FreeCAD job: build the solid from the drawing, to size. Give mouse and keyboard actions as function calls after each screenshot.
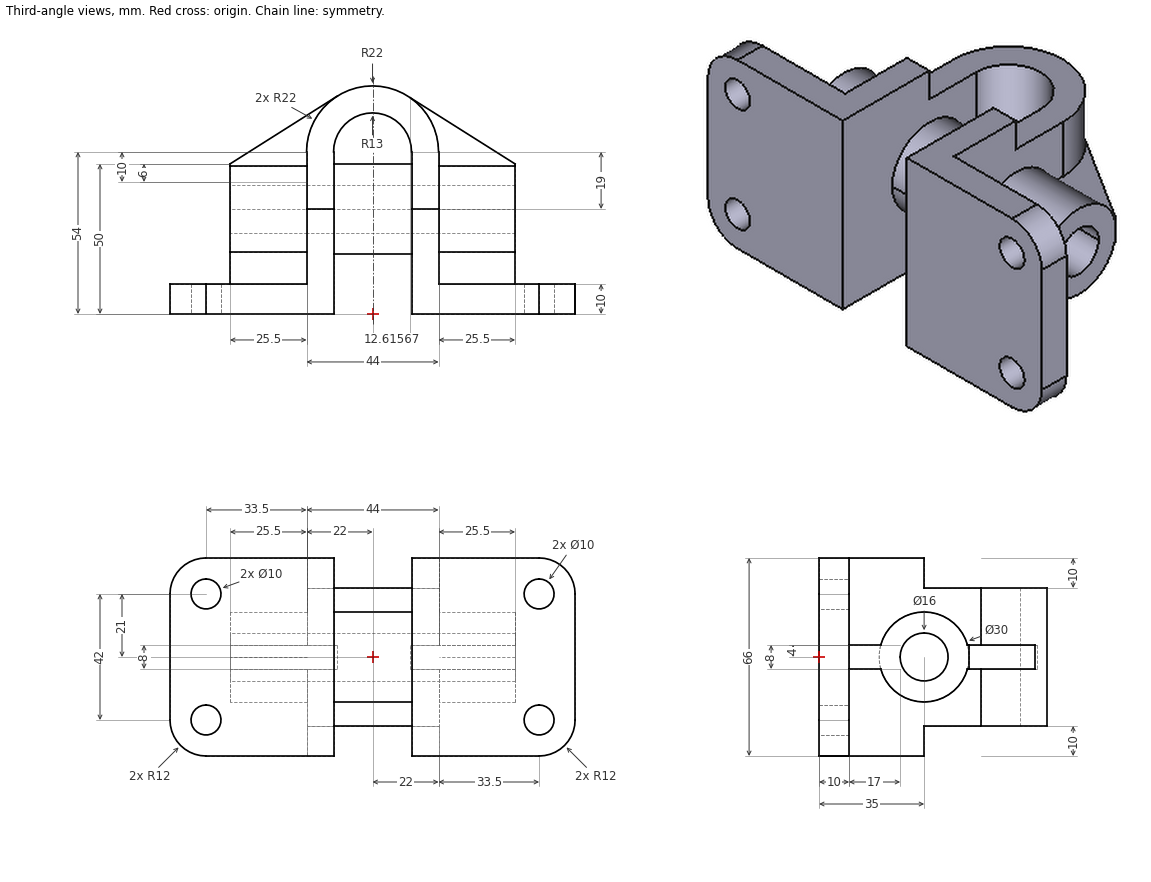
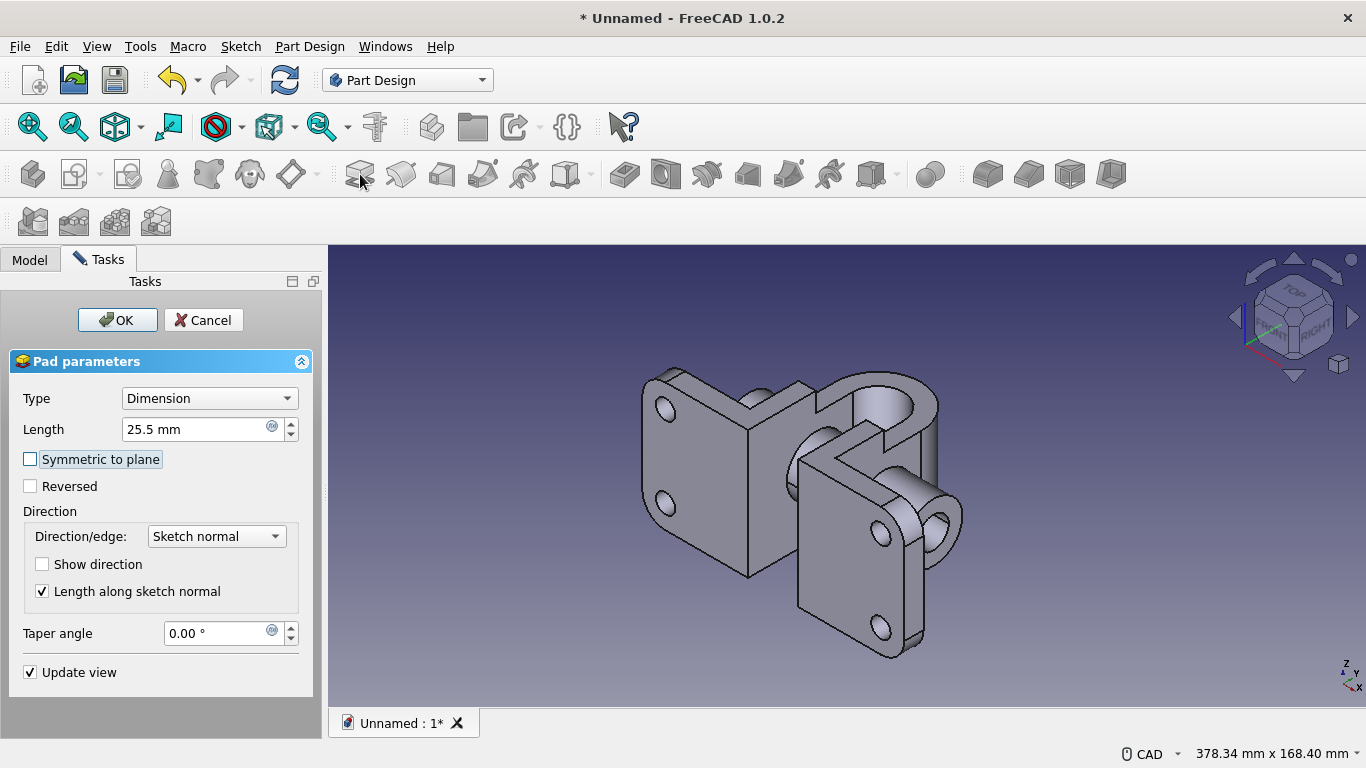
click(118, 320)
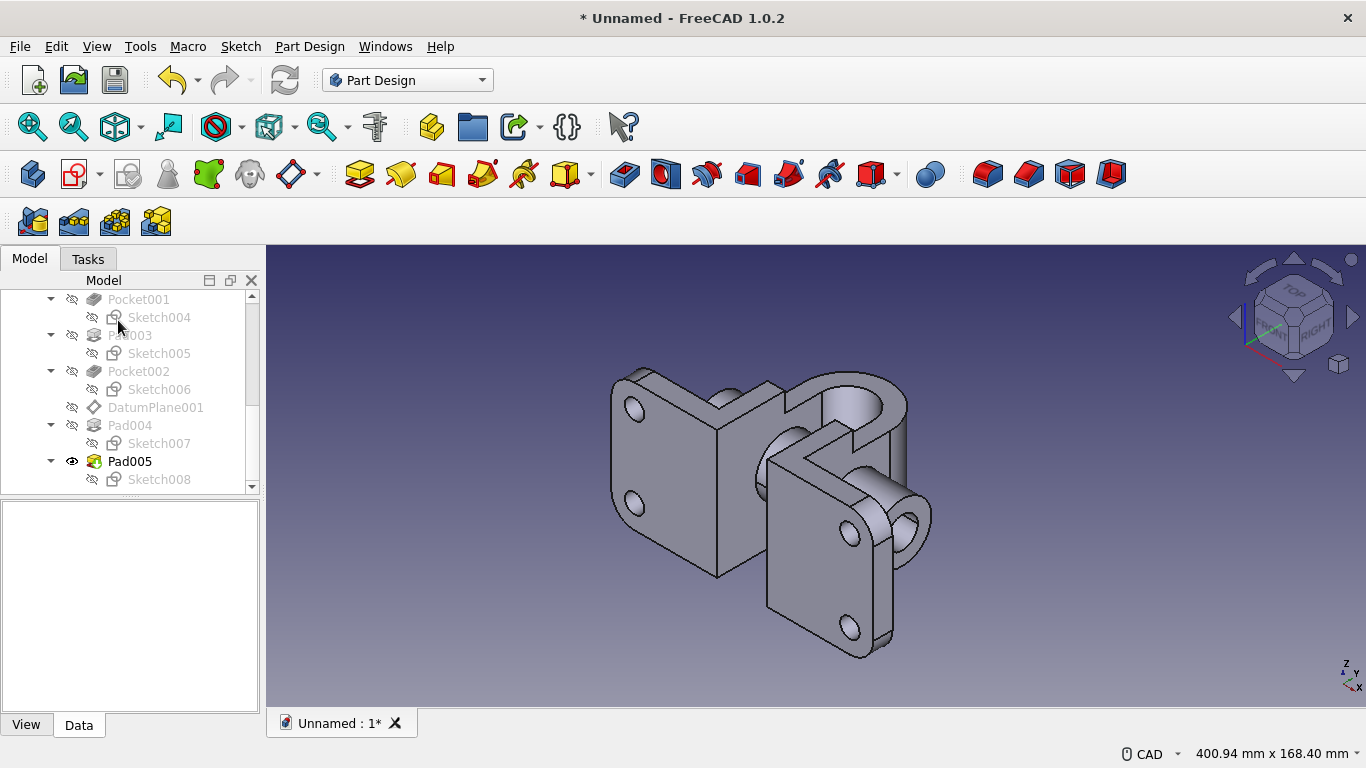
click(919, 503)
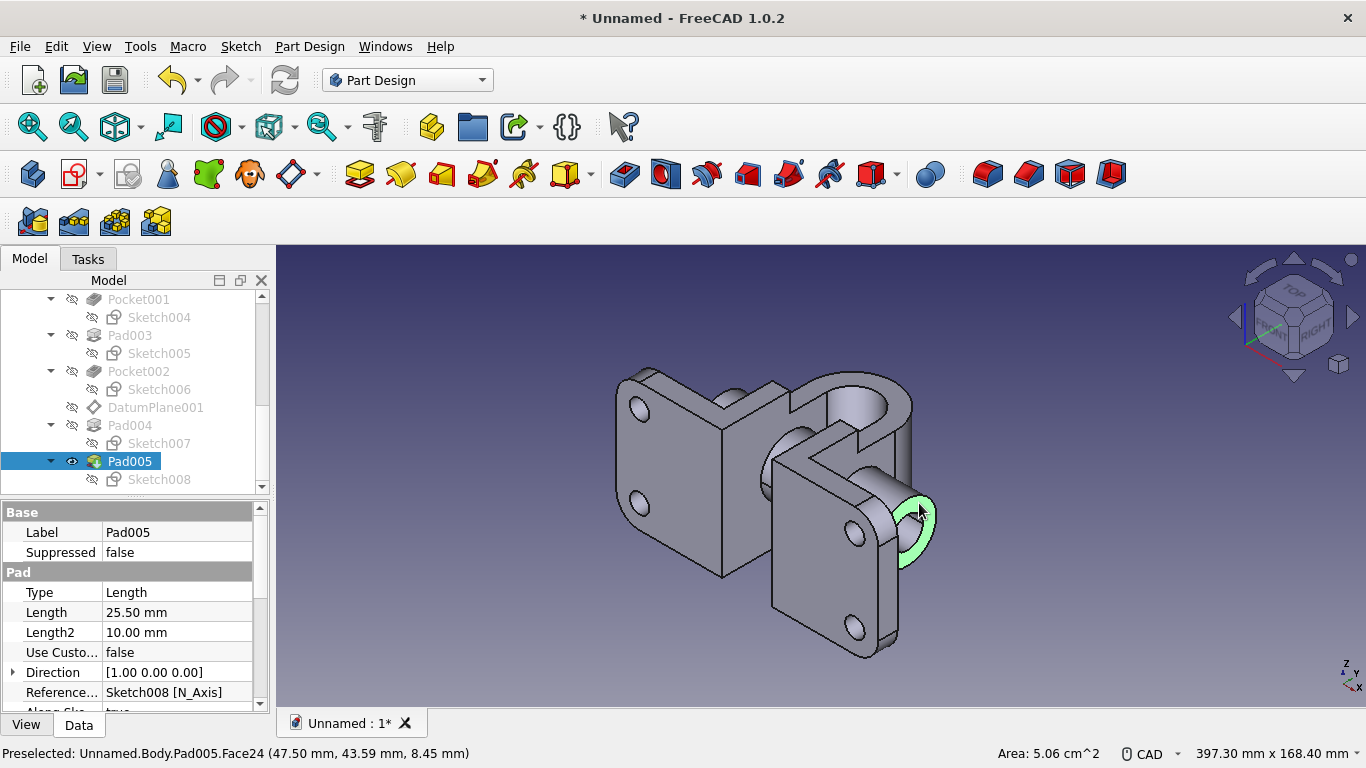
click(74, 174)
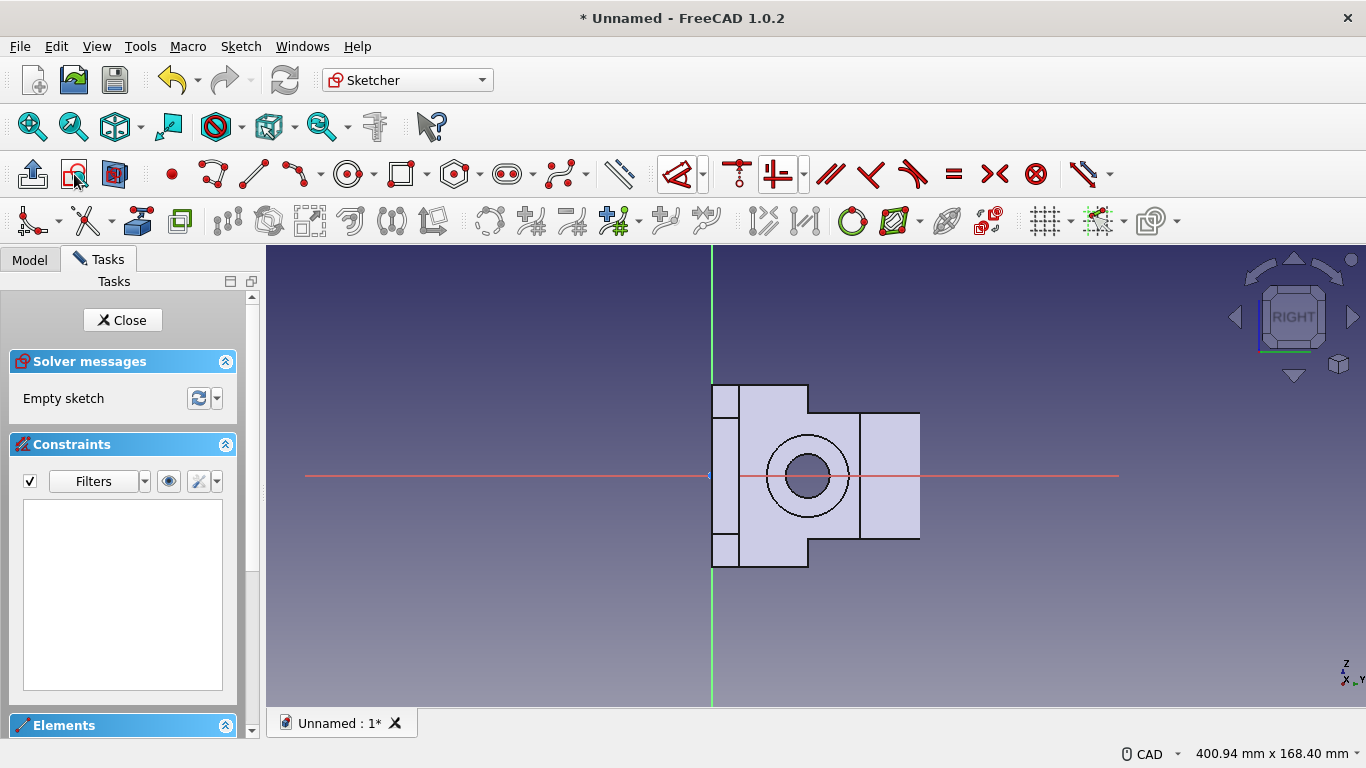
click(115, 174)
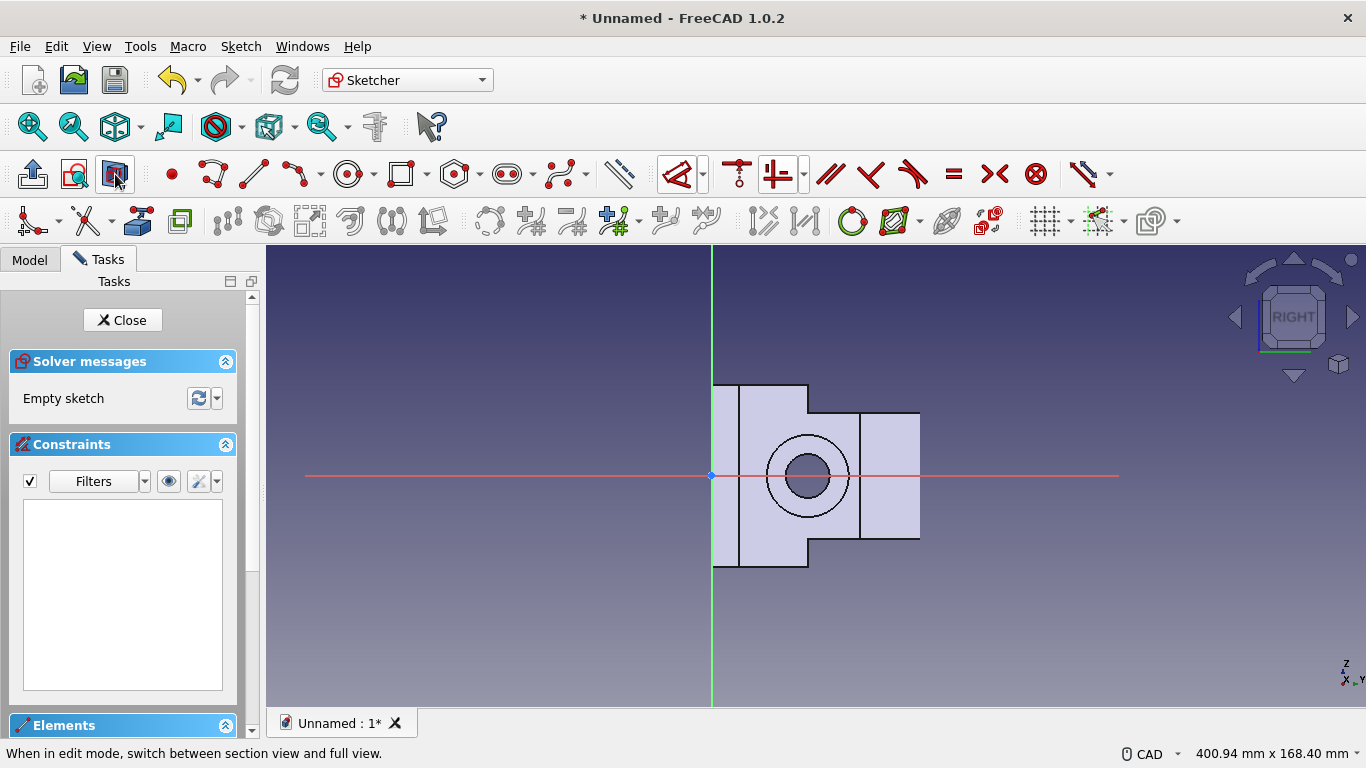
scroll(749, 476, up, 11)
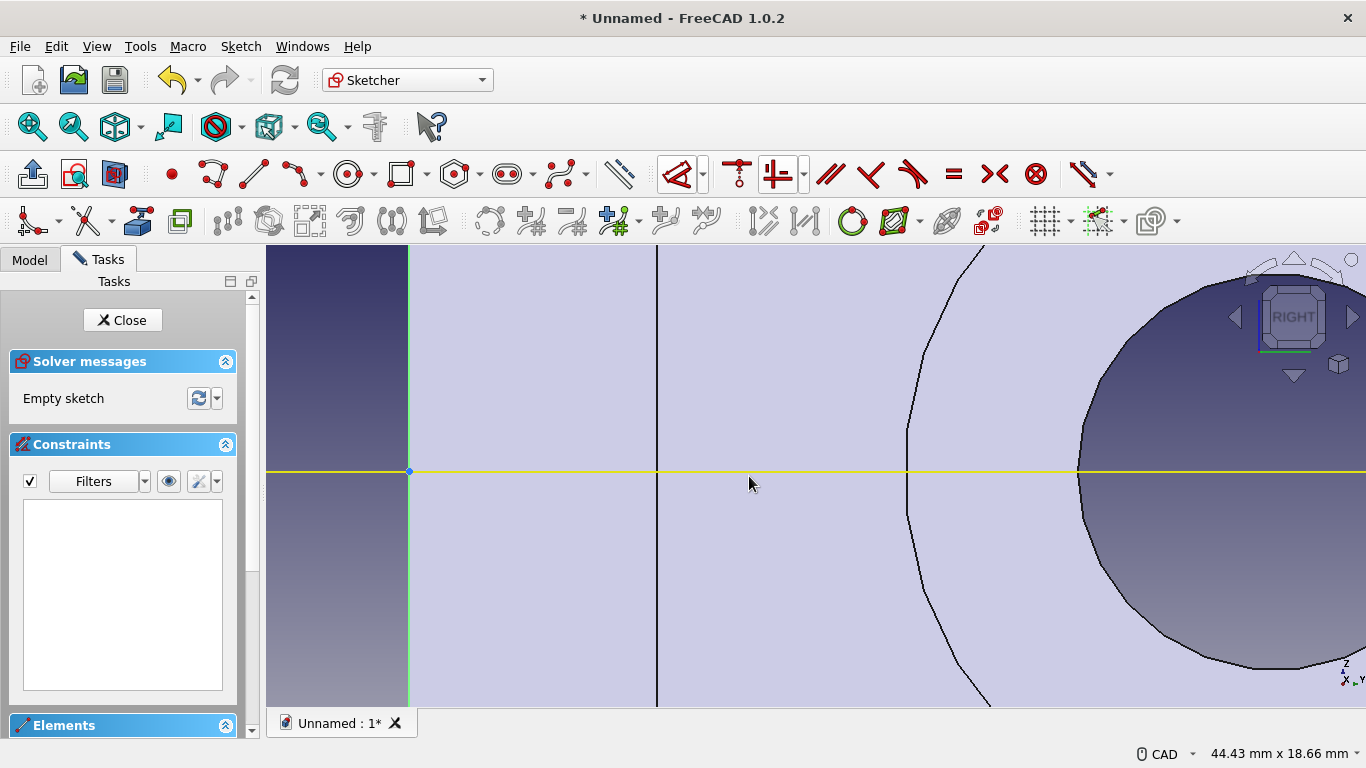
click(400, 174)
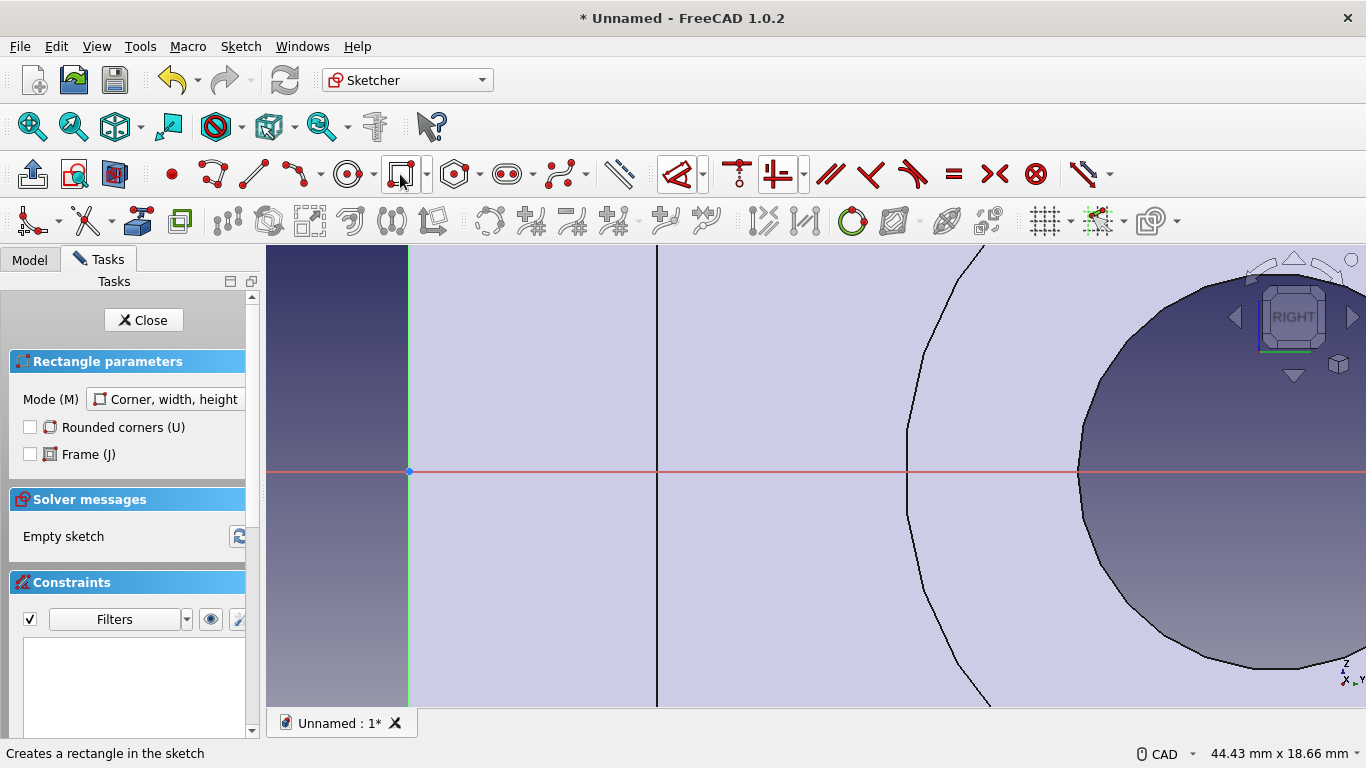
click(657, 373)
move(1078, 571)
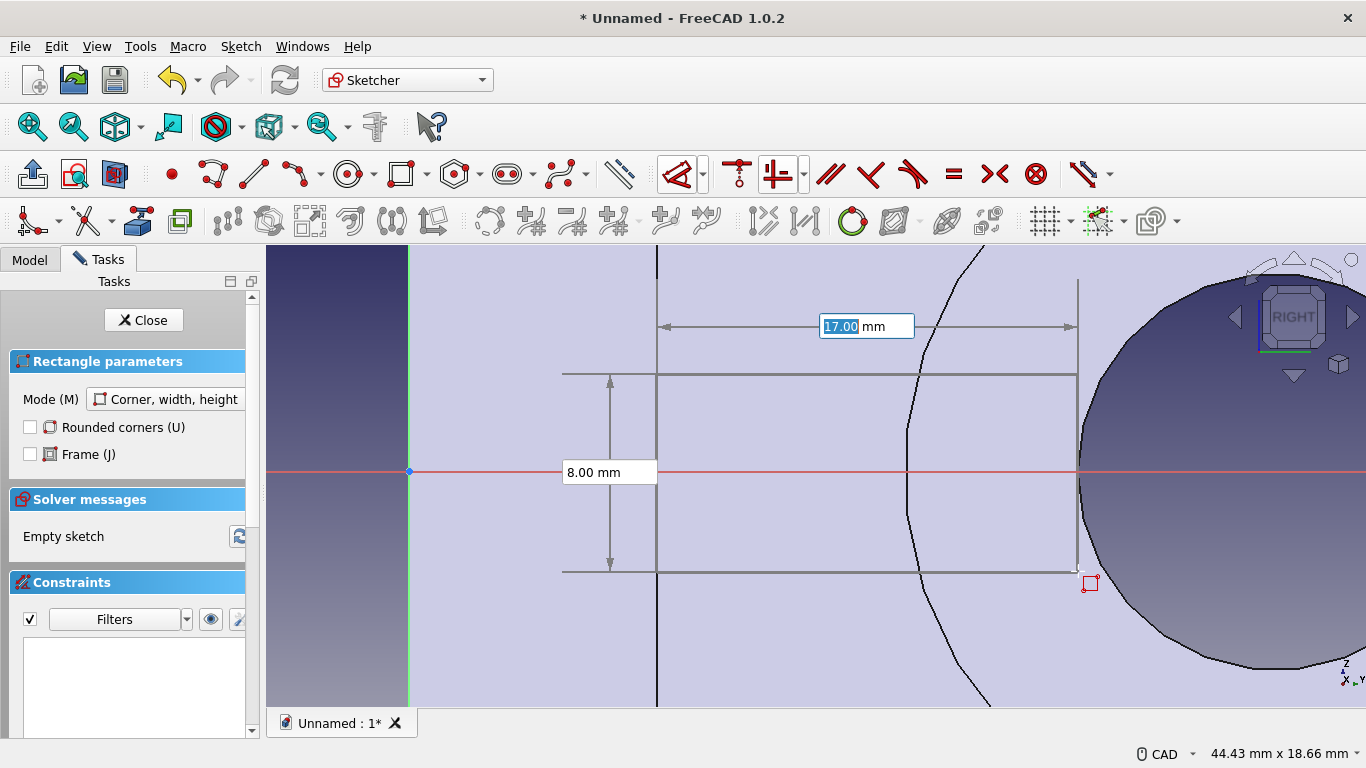
text(17)
key(Tab)
text(8)
key(Return)
key(Escape)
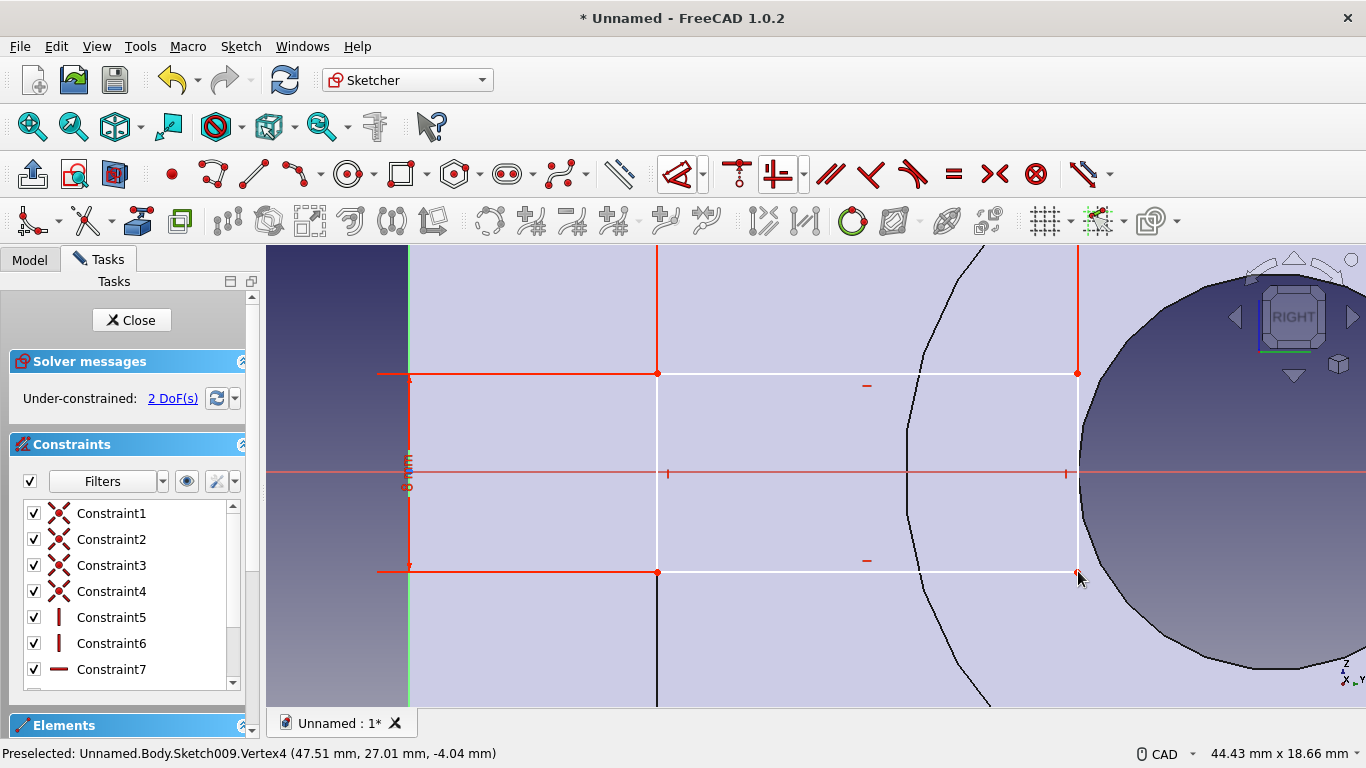
click(657, 374)